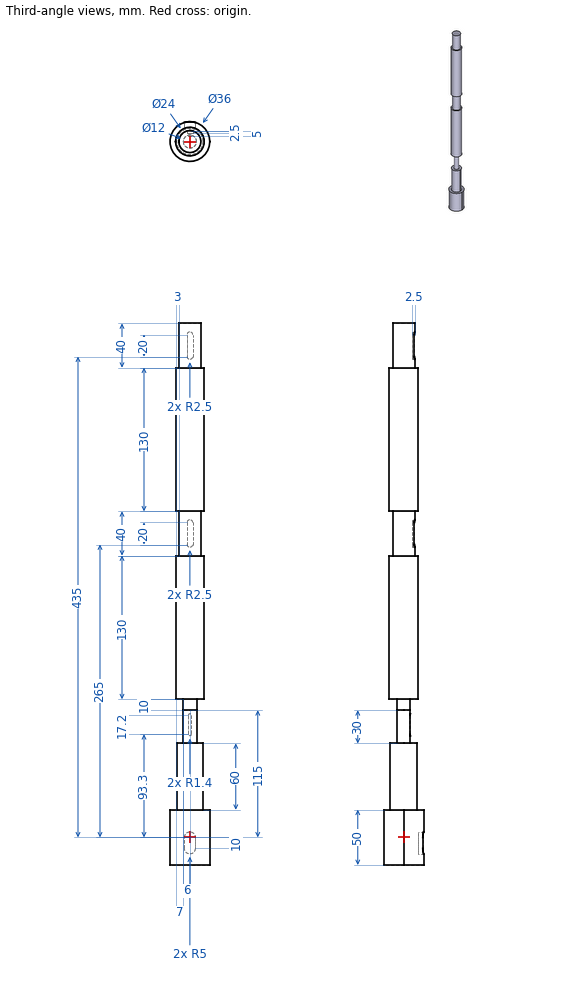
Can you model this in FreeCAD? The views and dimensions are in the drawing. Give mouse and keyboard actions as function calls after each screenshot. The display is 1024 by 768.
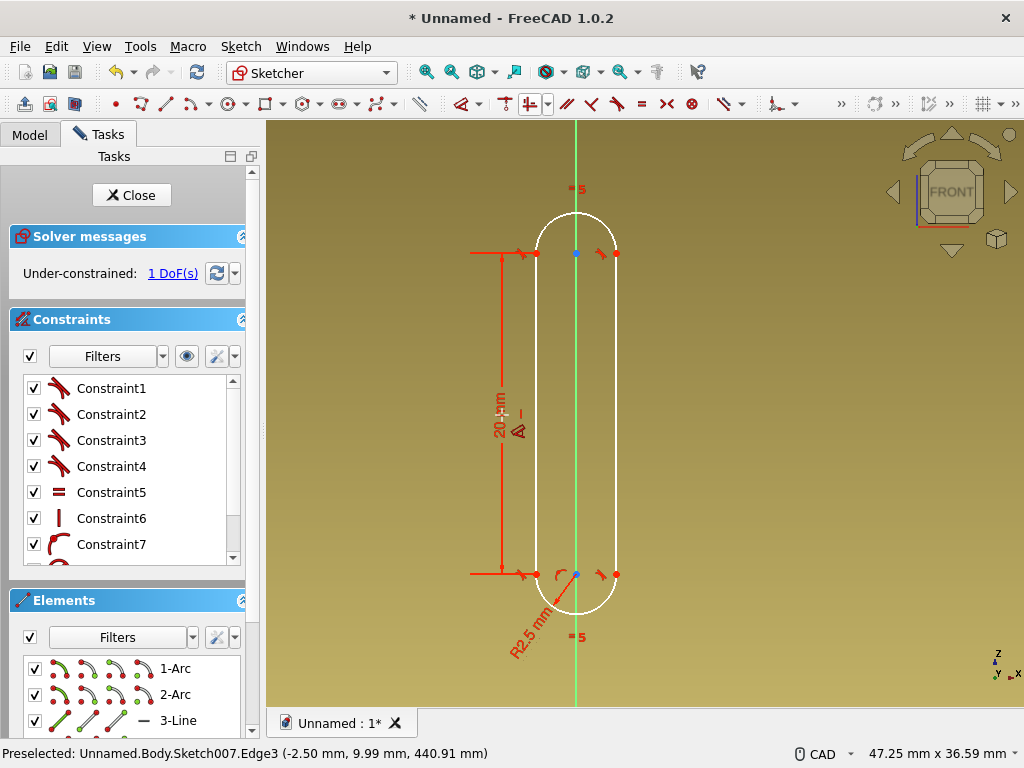
click(536, 574)
click(502, 602)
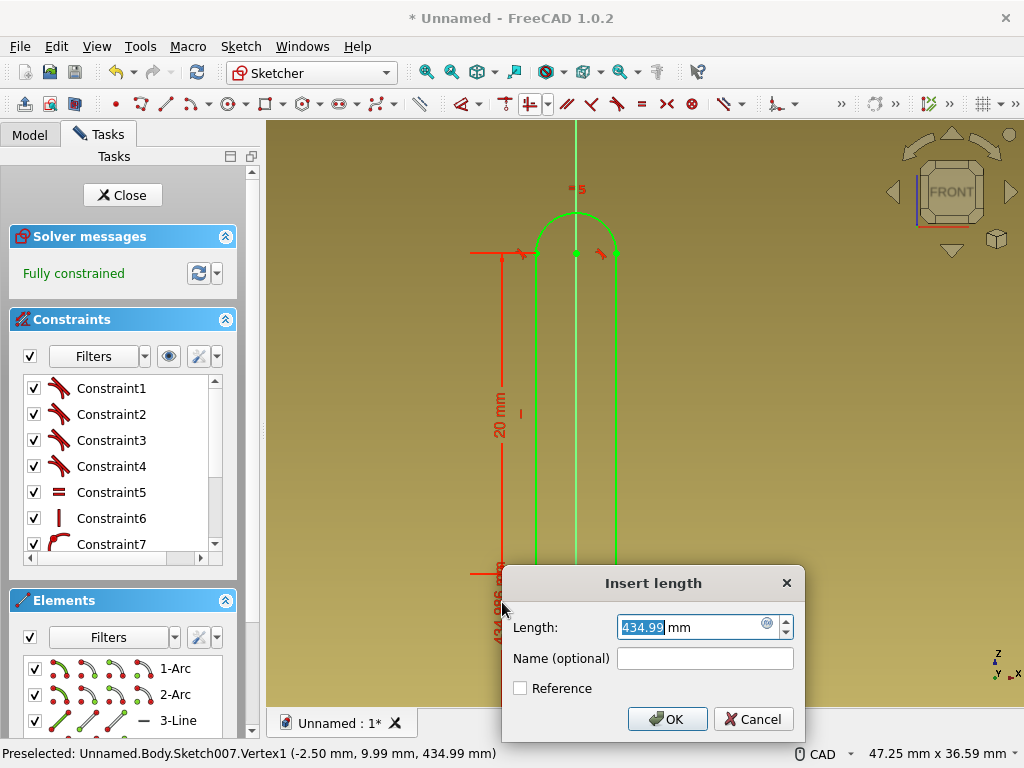
text(435)
key(Return)
key(Escape)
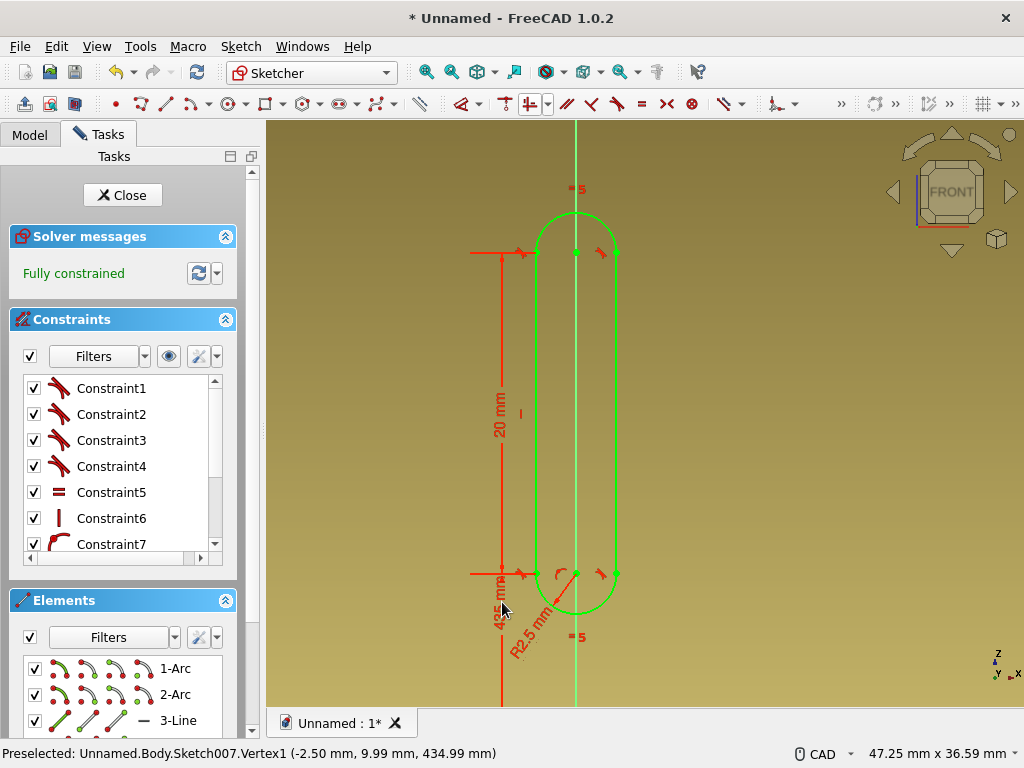
click(123, 195)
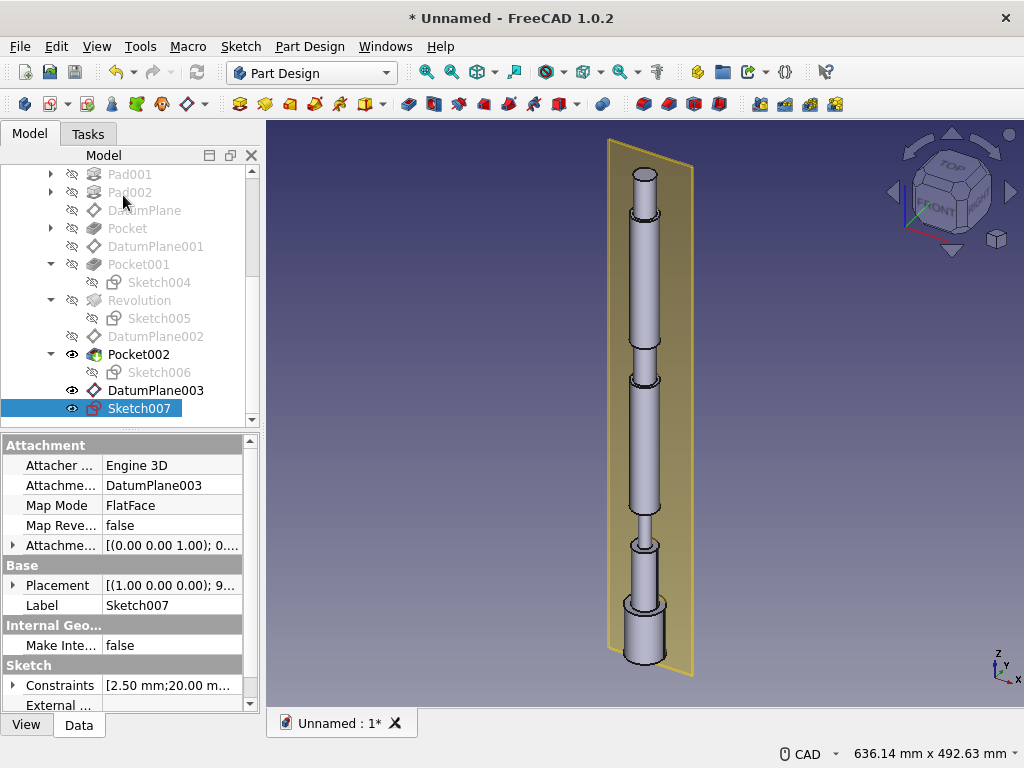
click(409, 104)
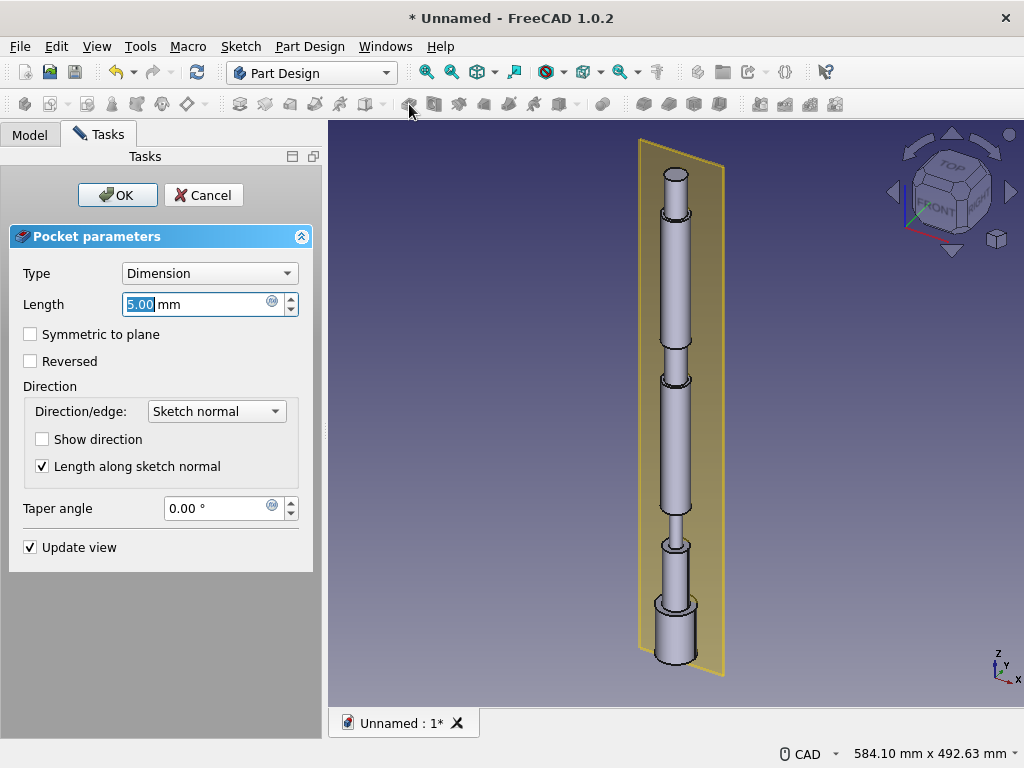
text(2.5)
key(Tab)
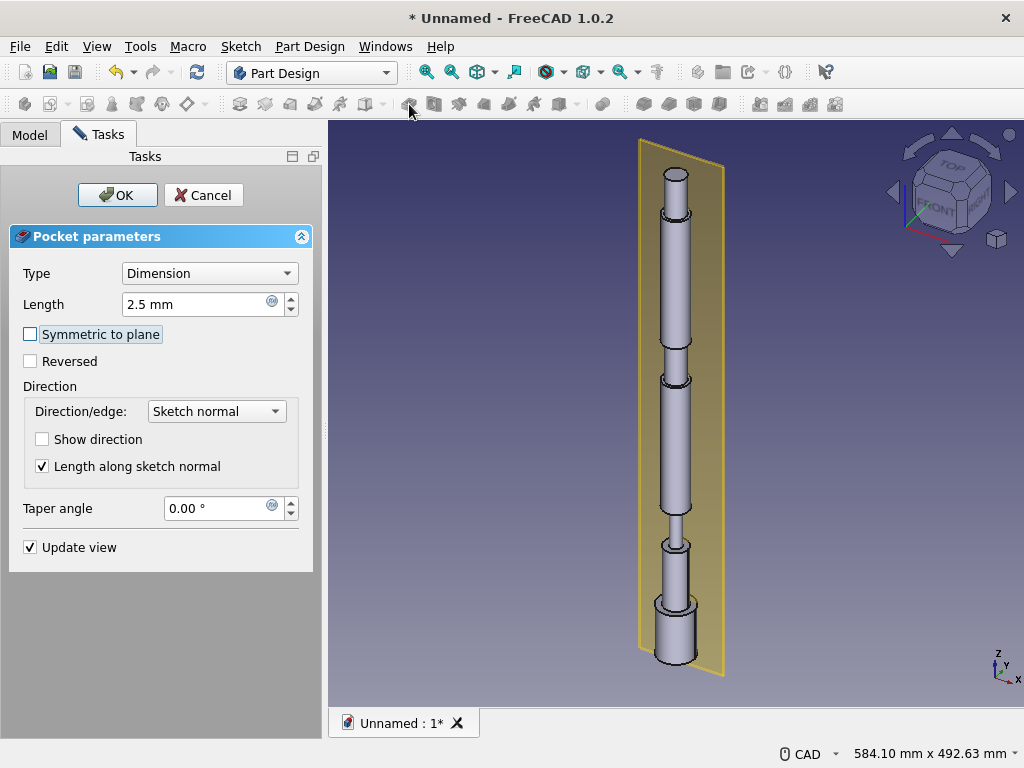
click(31, 361)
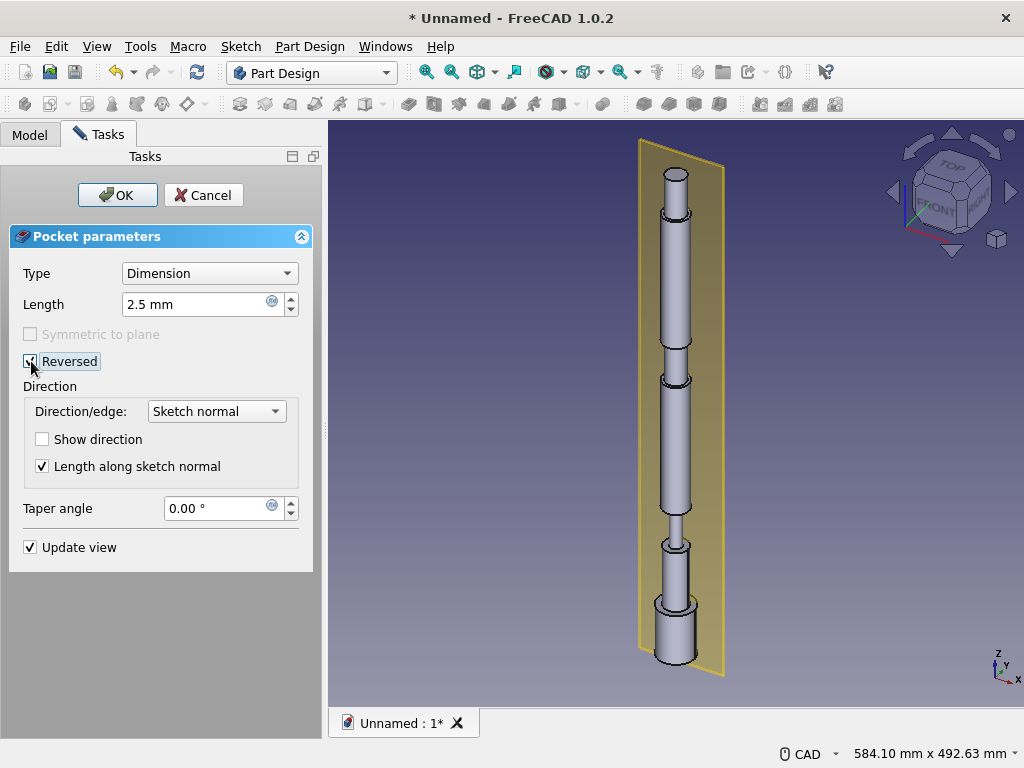
click(118, 195)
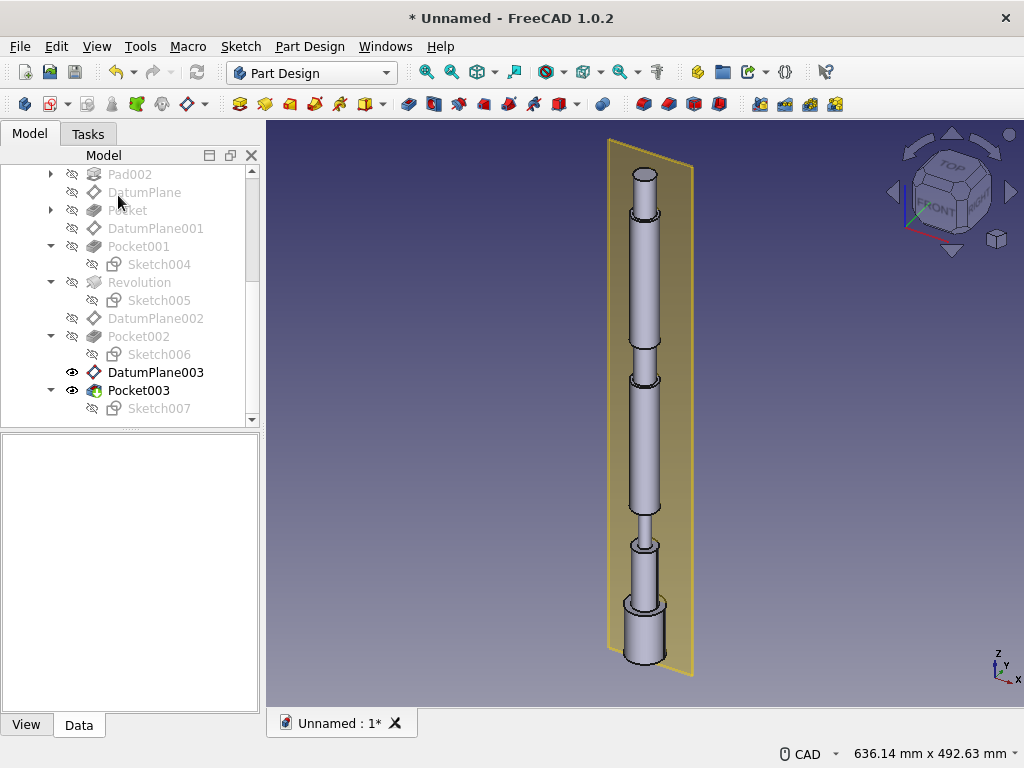
click(117, 372)
key(space)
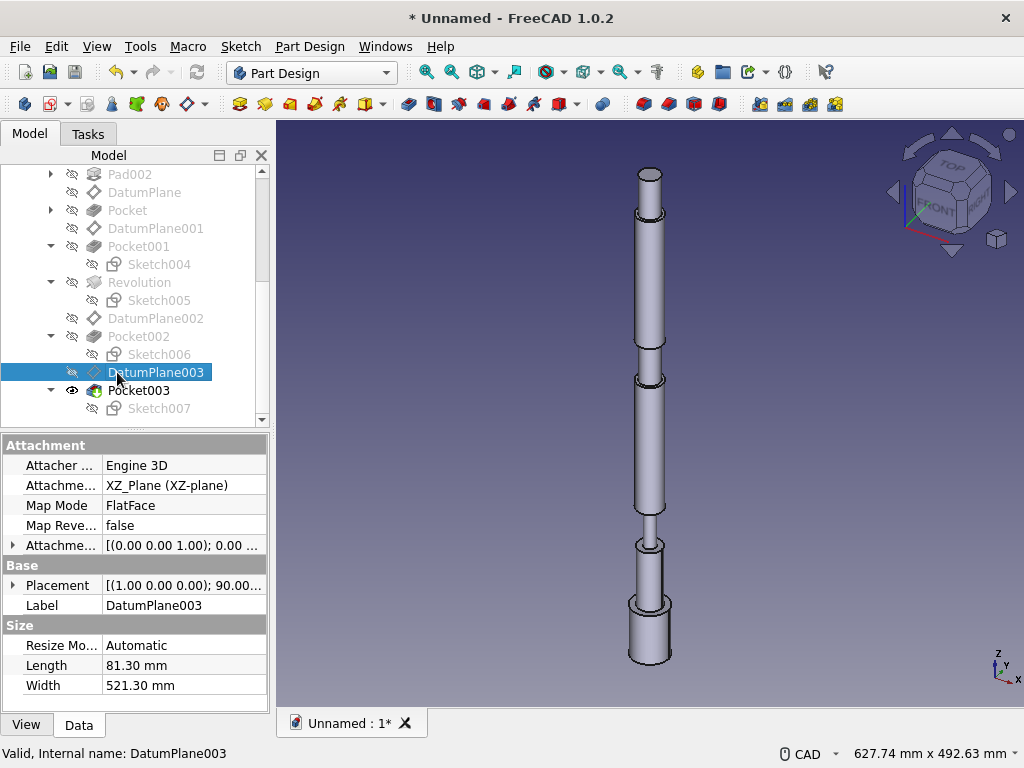
key(0)